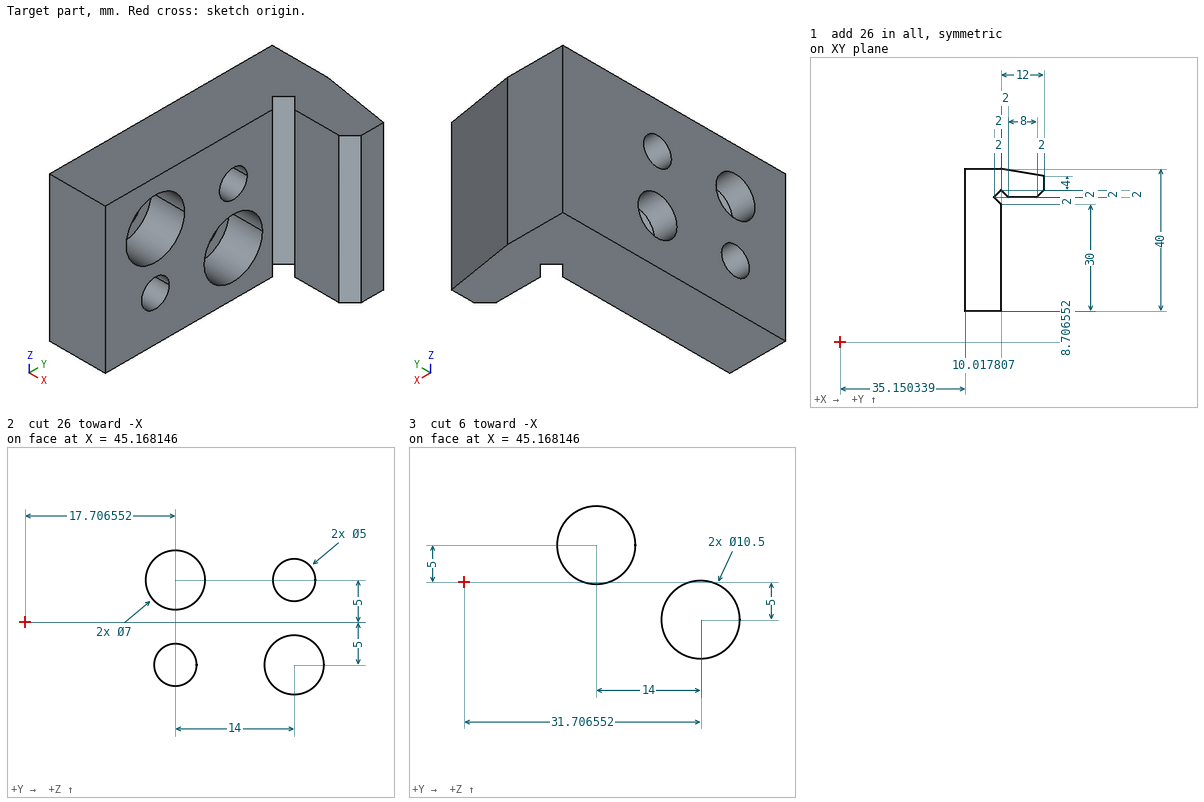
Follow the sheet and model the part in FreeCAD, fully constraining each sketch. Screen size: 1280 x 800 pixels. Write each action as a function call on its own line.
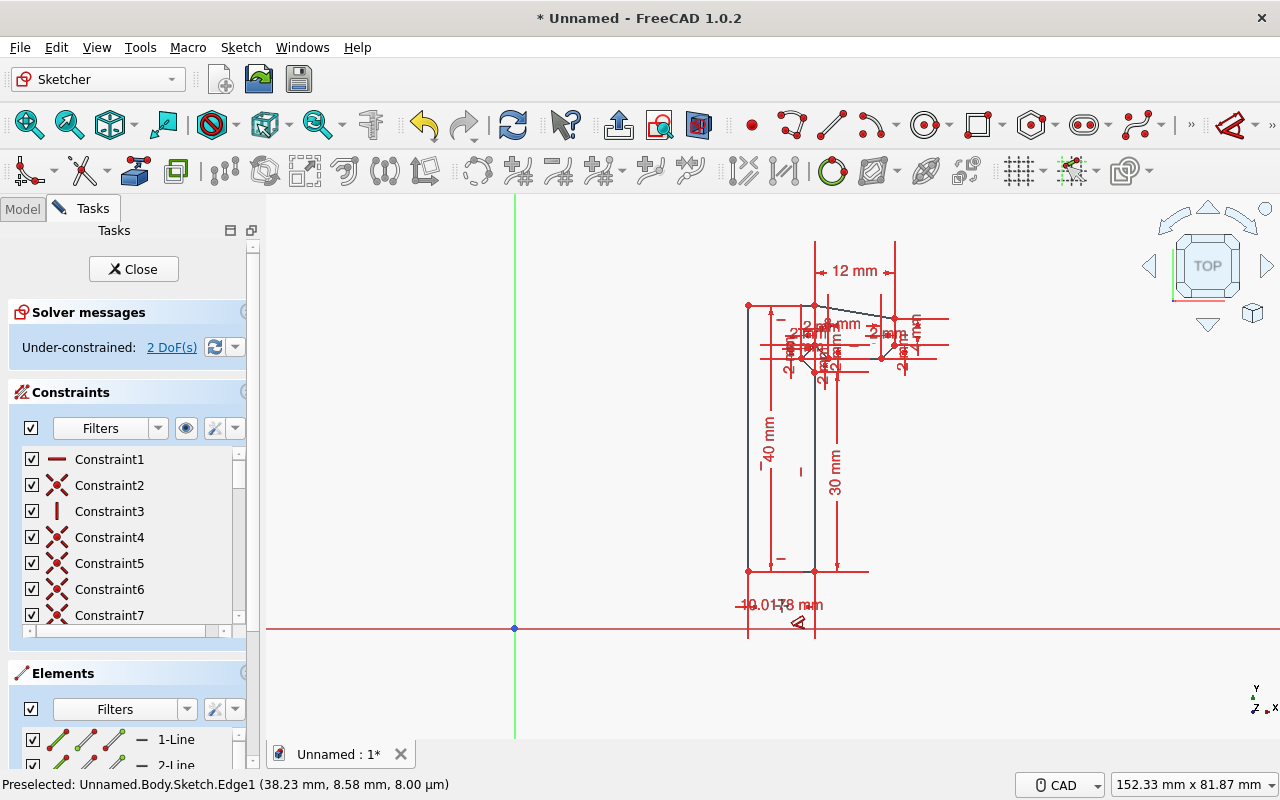
click(748, 572)
click(481, 600)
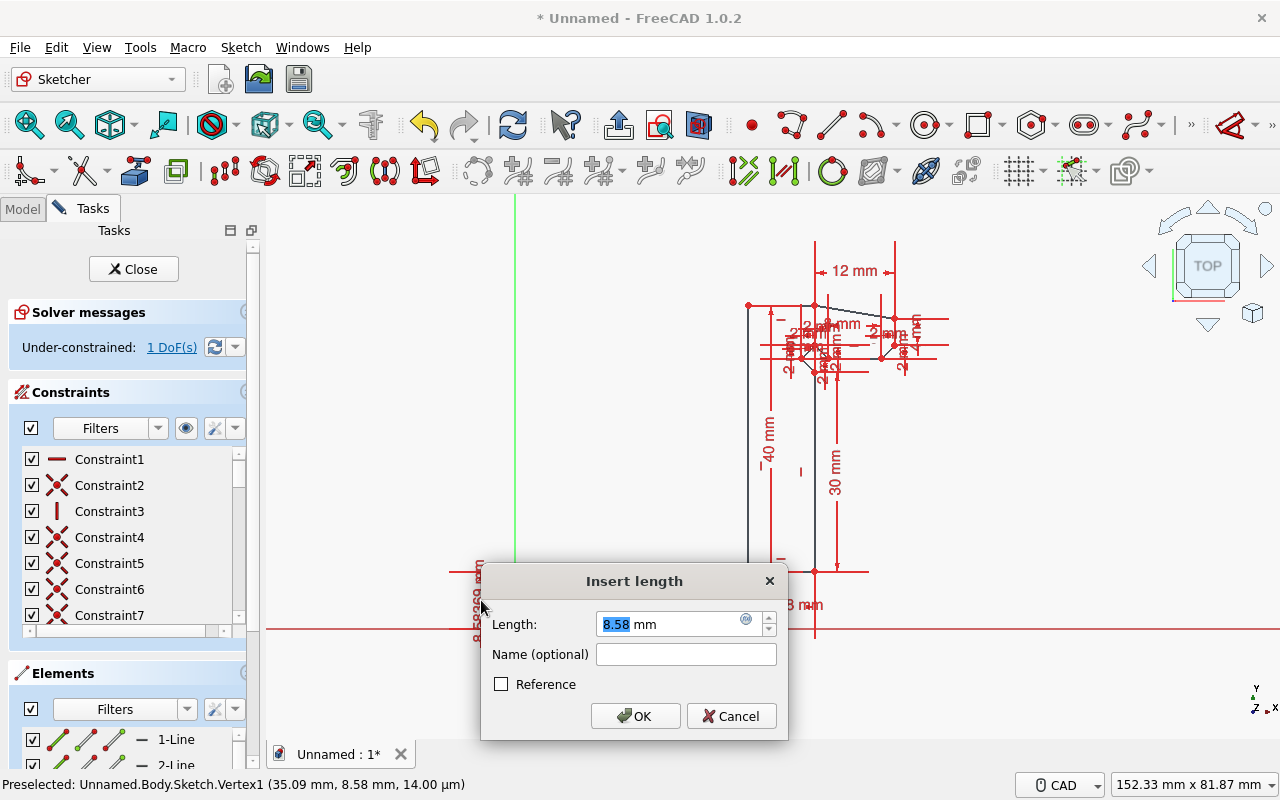
text(8.706552)
key(Return)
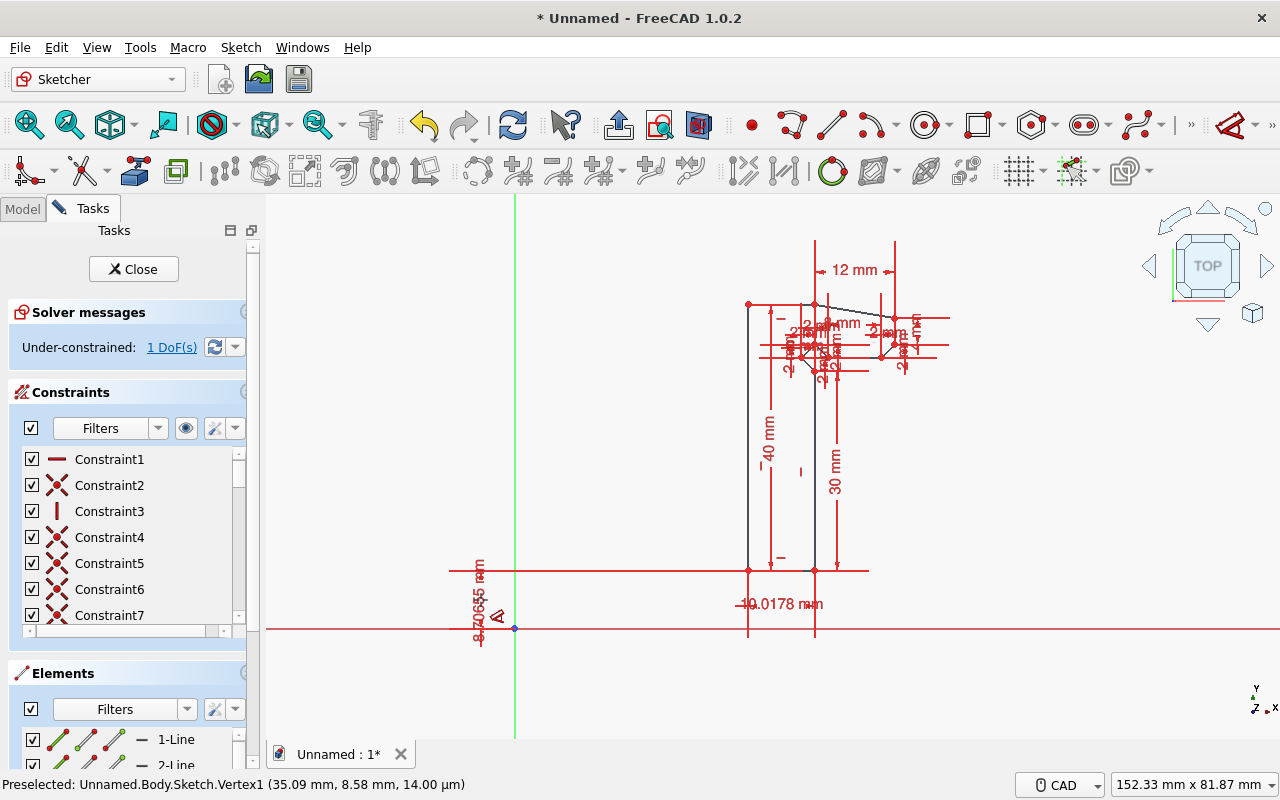
click(748, 571)
click(631, 663)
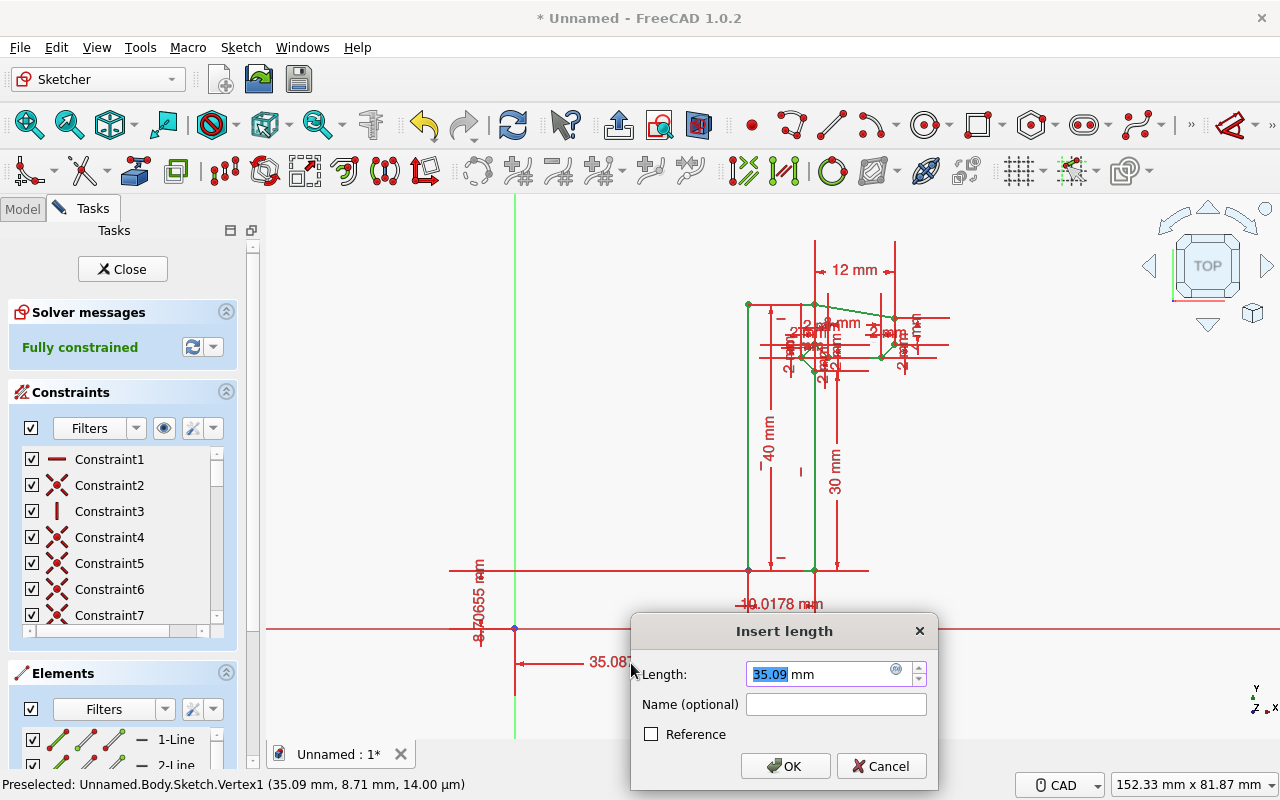
text(35.150339)
key(Return)
key(Escape)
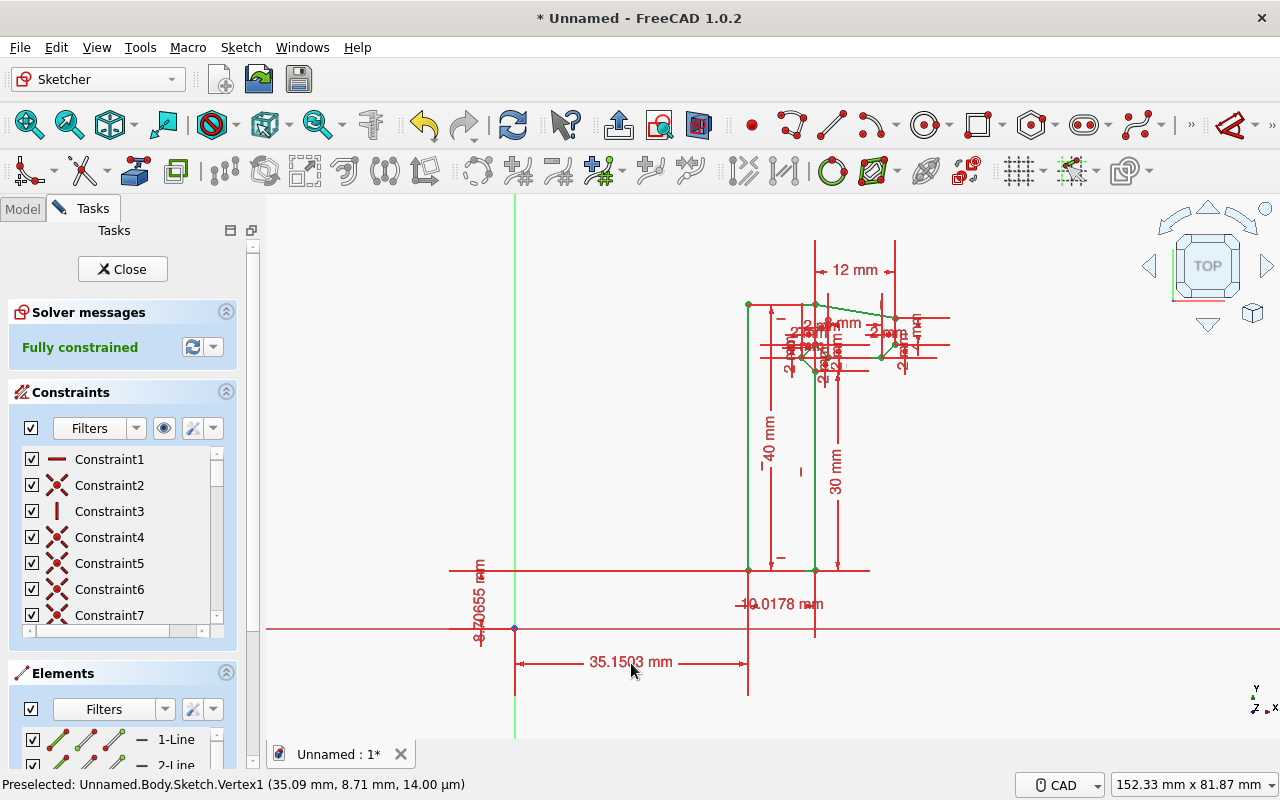
click(123, 269)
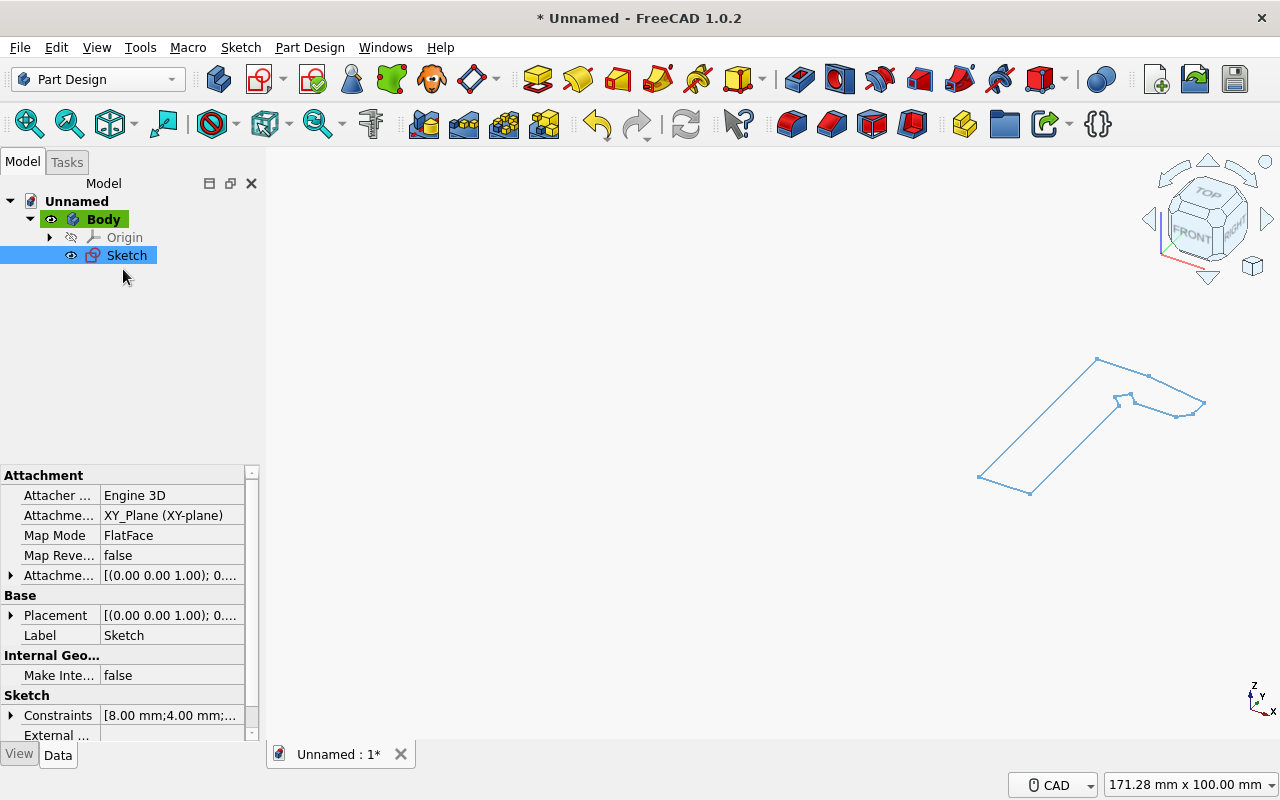
click(538, 80)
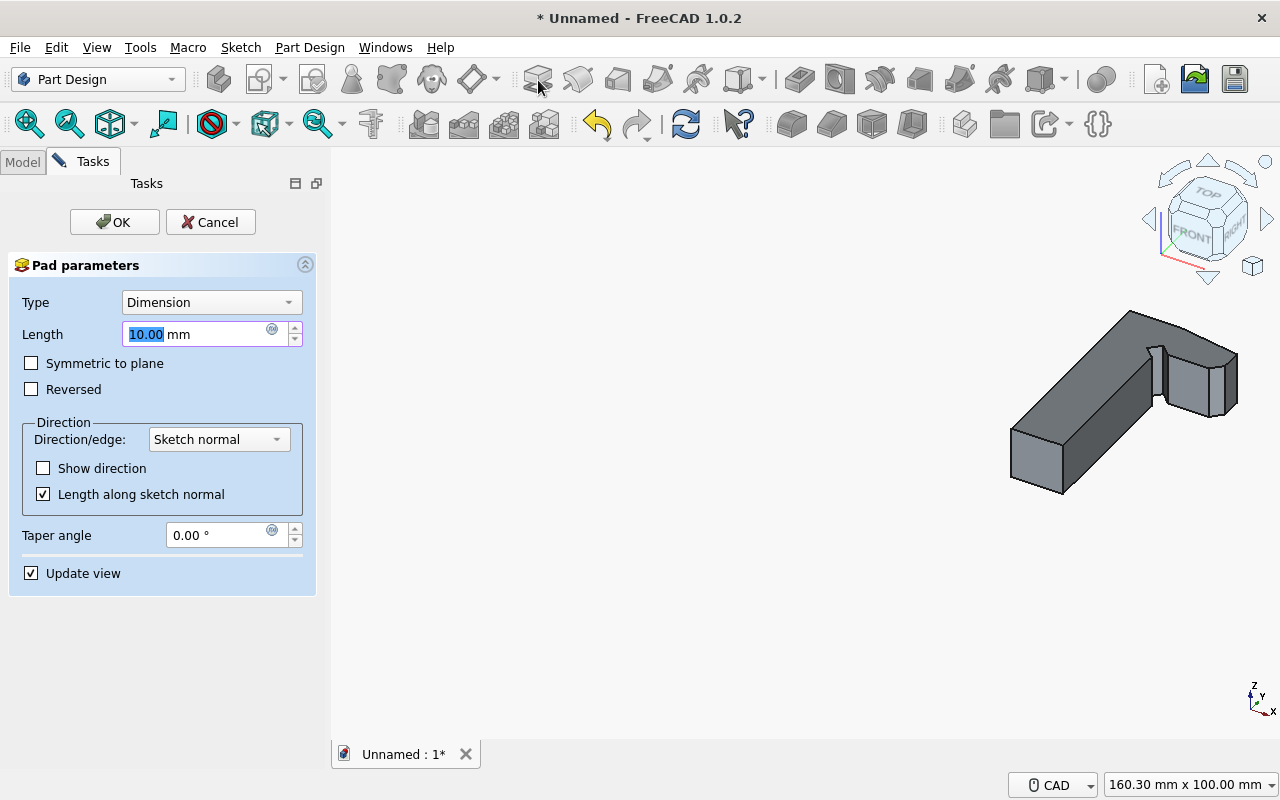
text(26)
key(Tab)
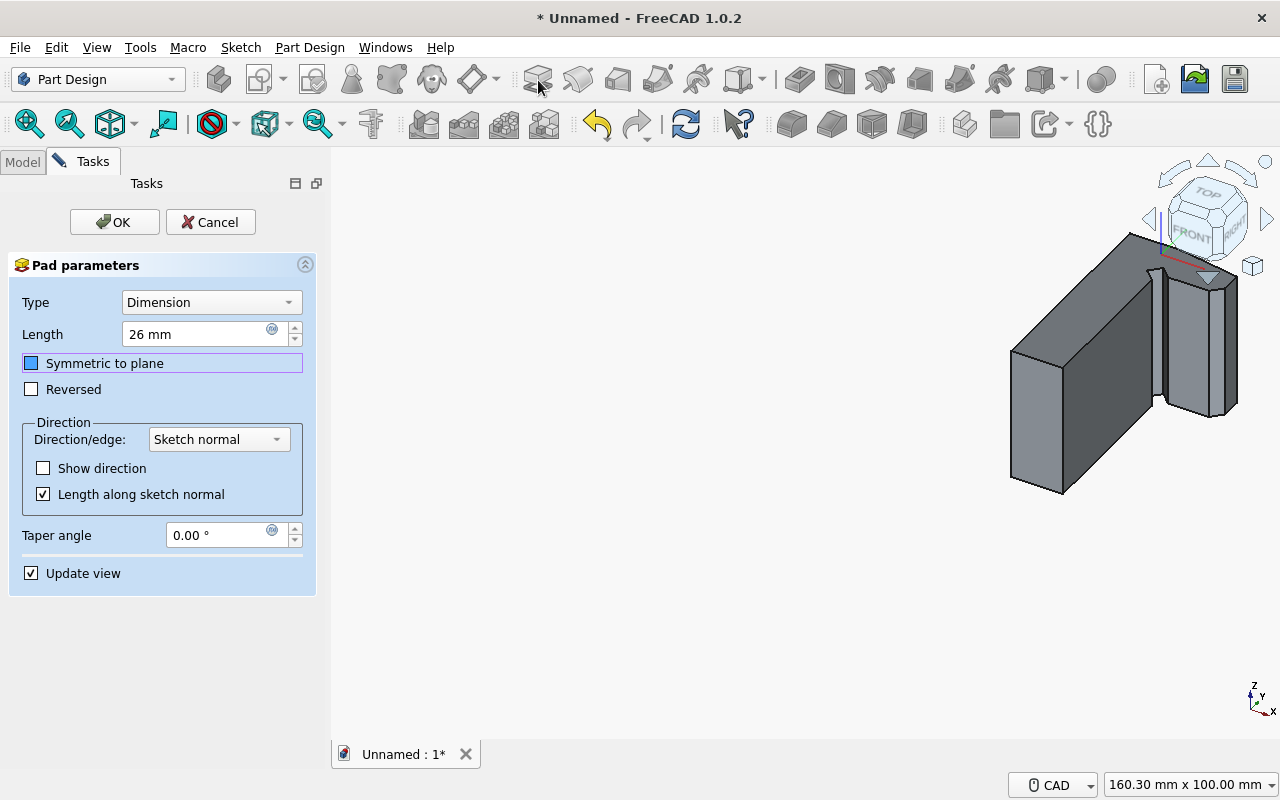
click(30, 363)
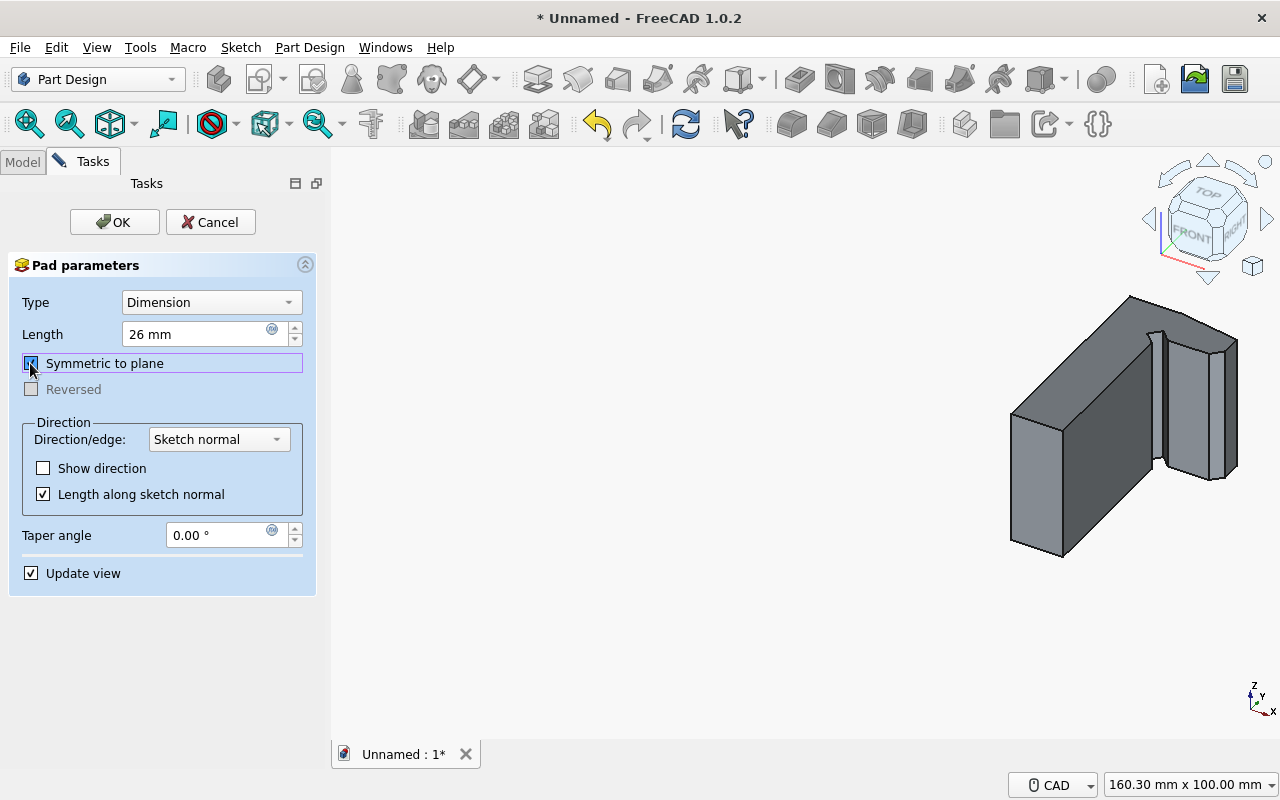
click(115, 222)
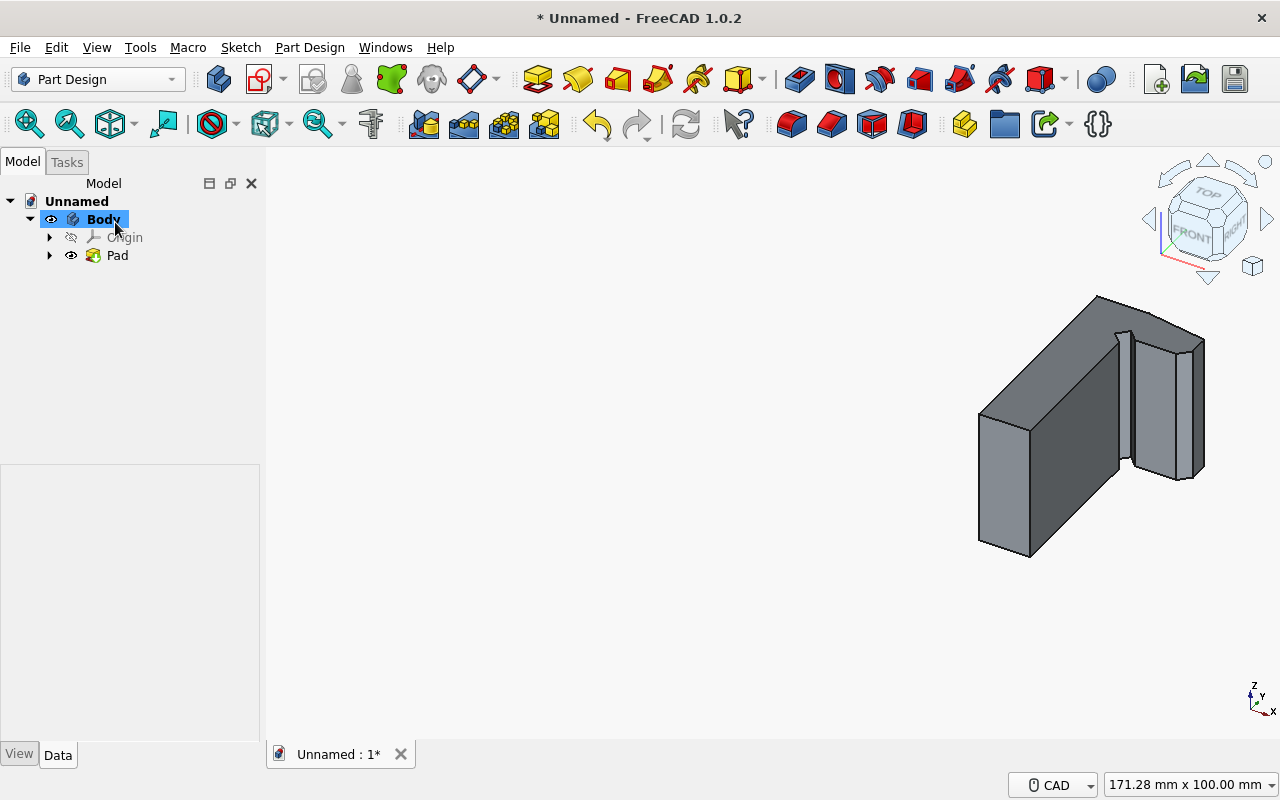
click(1075, 449)